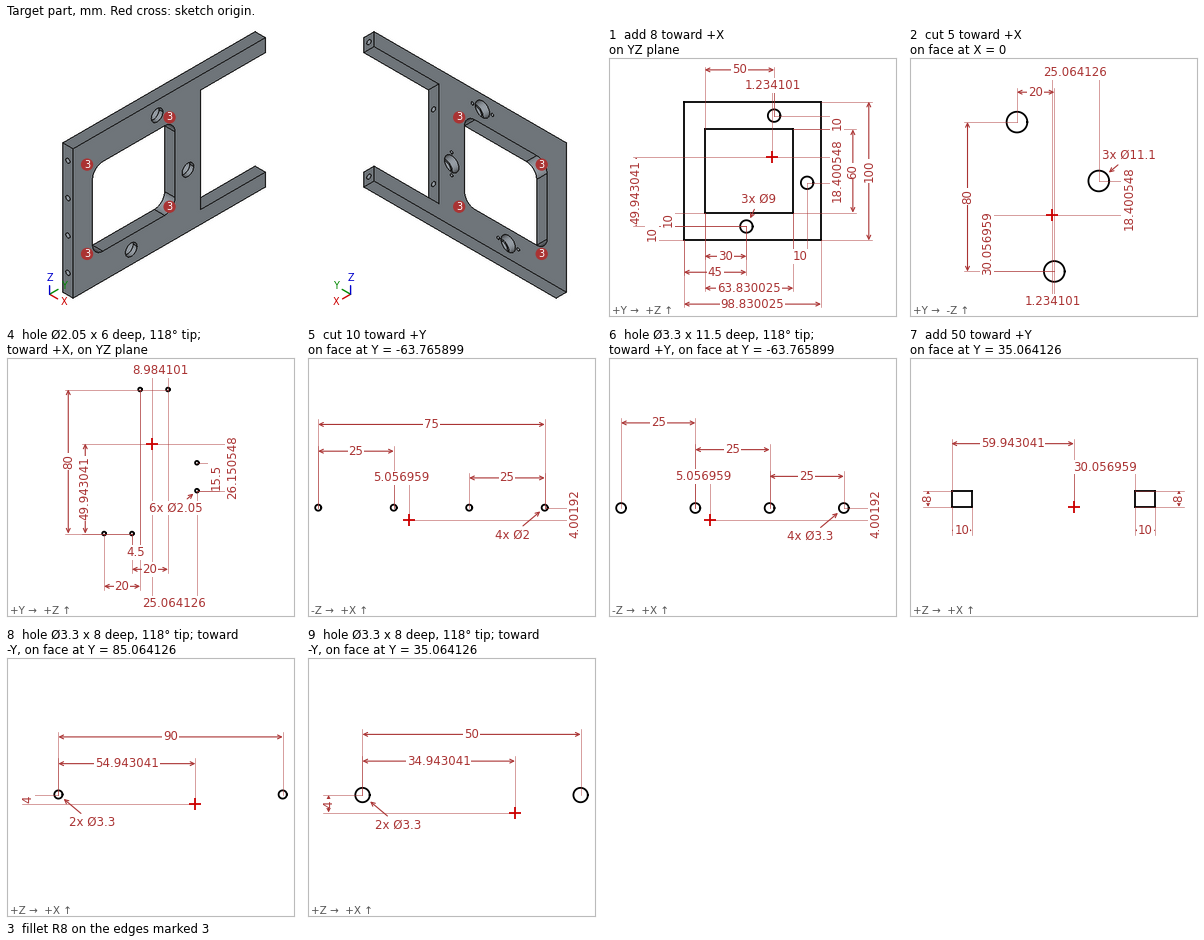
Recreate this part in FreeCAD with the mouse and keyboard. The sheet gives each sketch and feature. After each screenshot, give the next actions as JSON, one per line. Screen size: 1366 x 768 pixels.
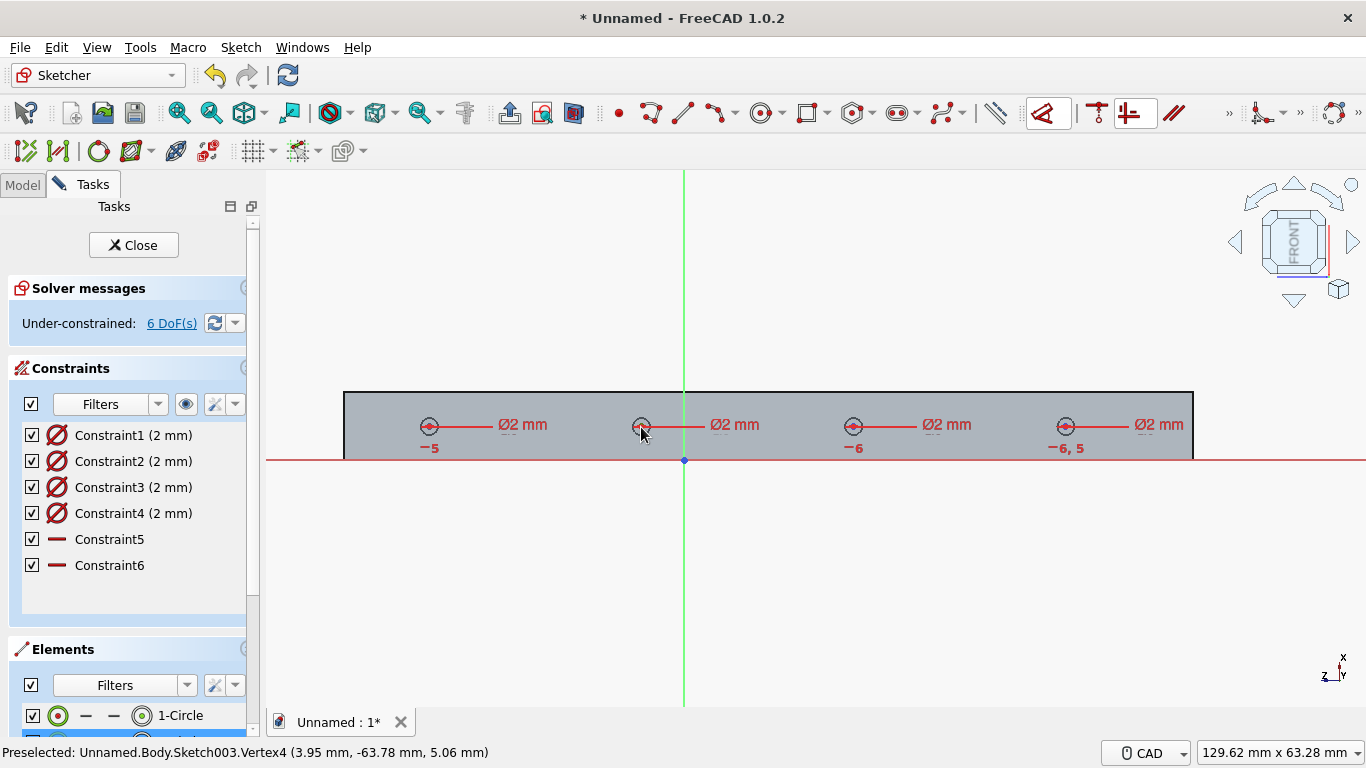
{"action": "left_click", "coordinate": [1152, 114]}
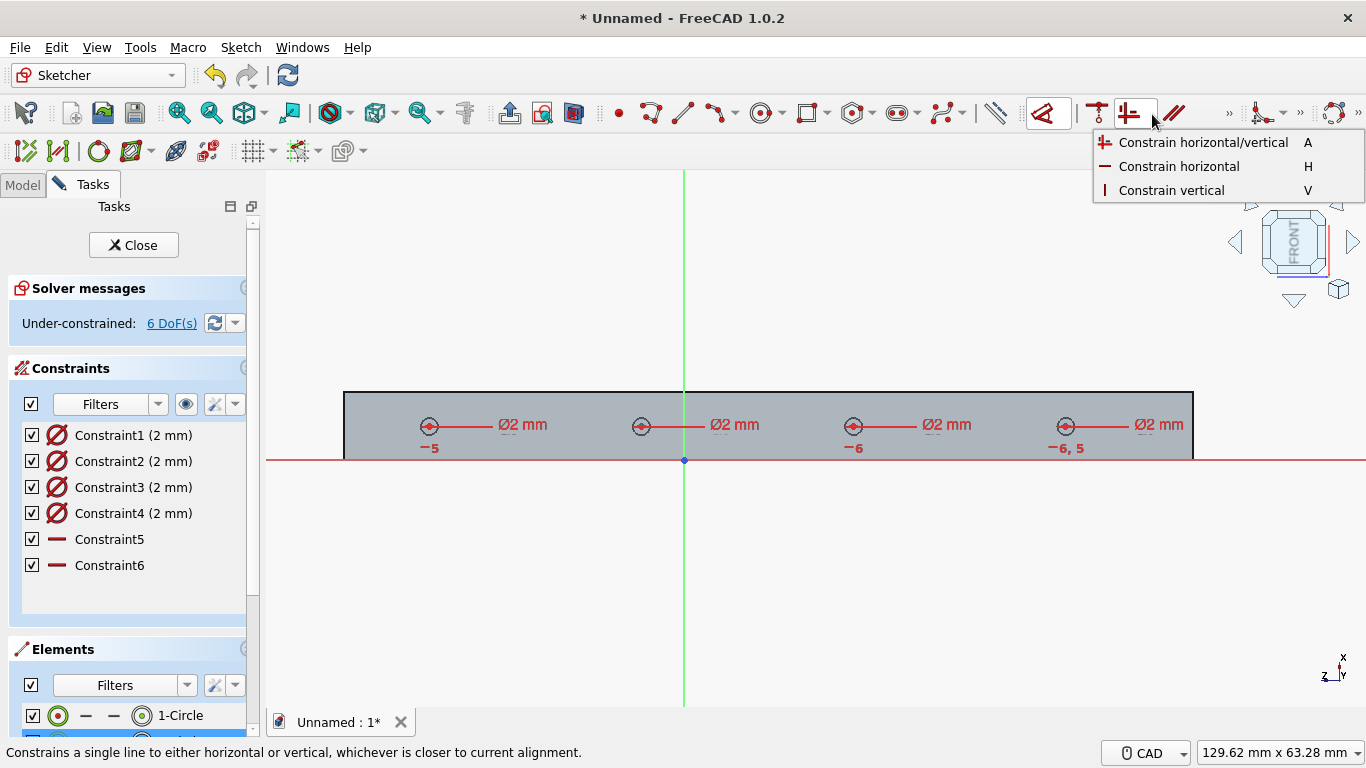
{"action": "left_click", "coordinate": [1229, 166]}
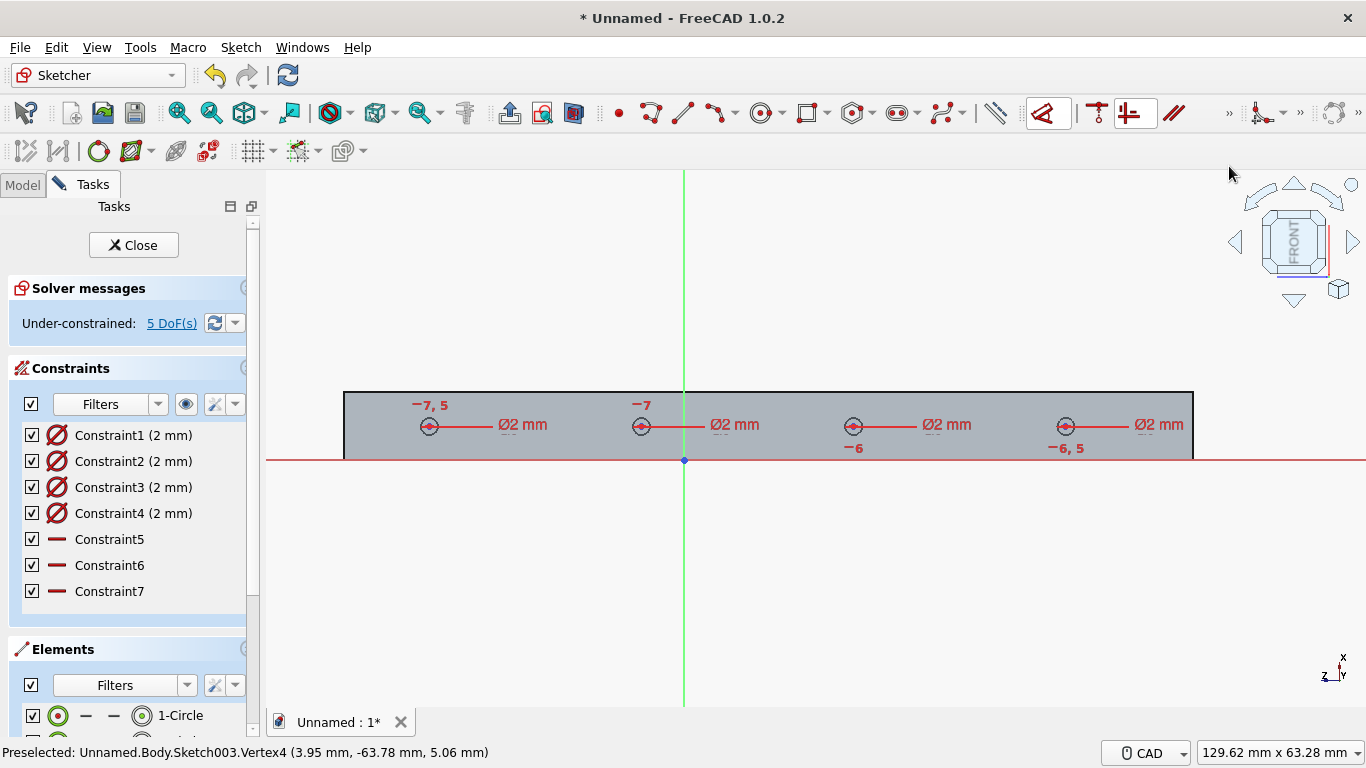
{"action": "left_click", "coordinate": [1066, 427]}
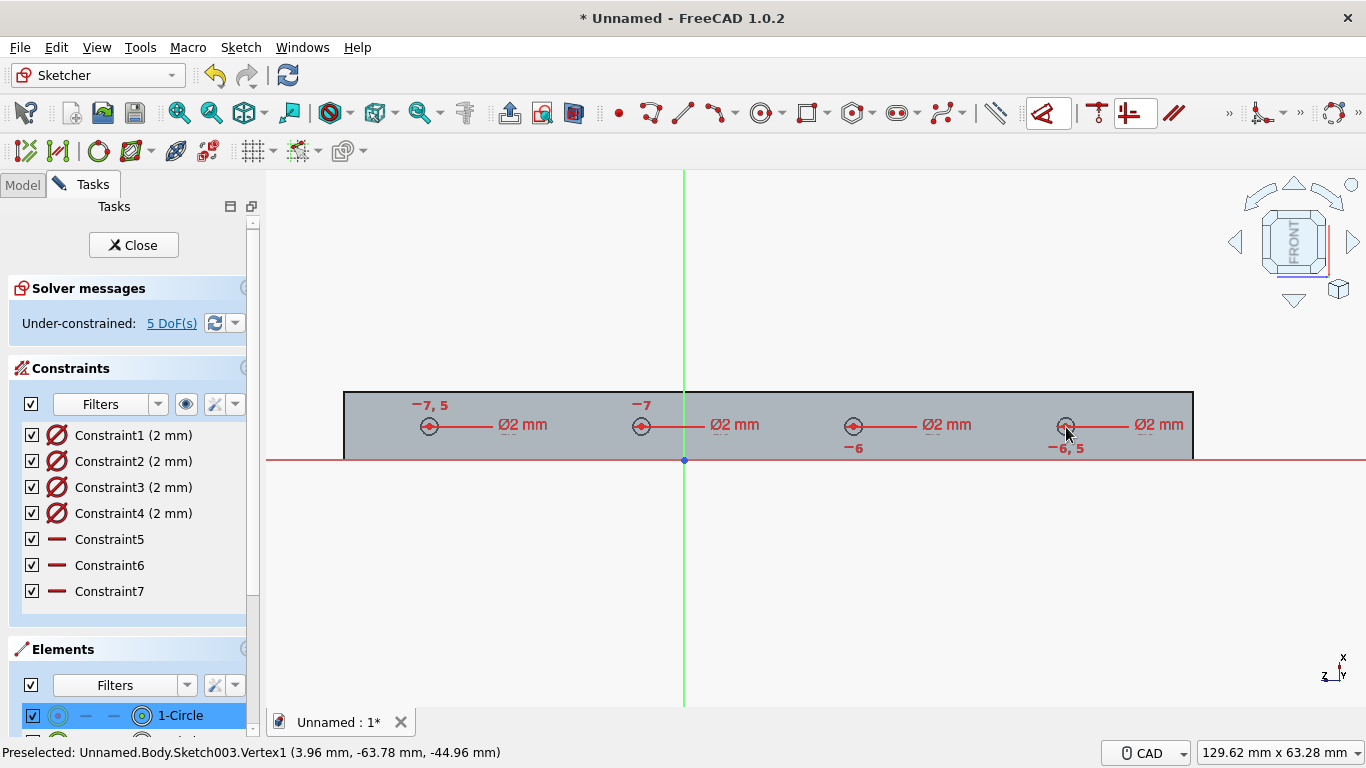
{"action": "left_click", "coordinate": [429, 427]}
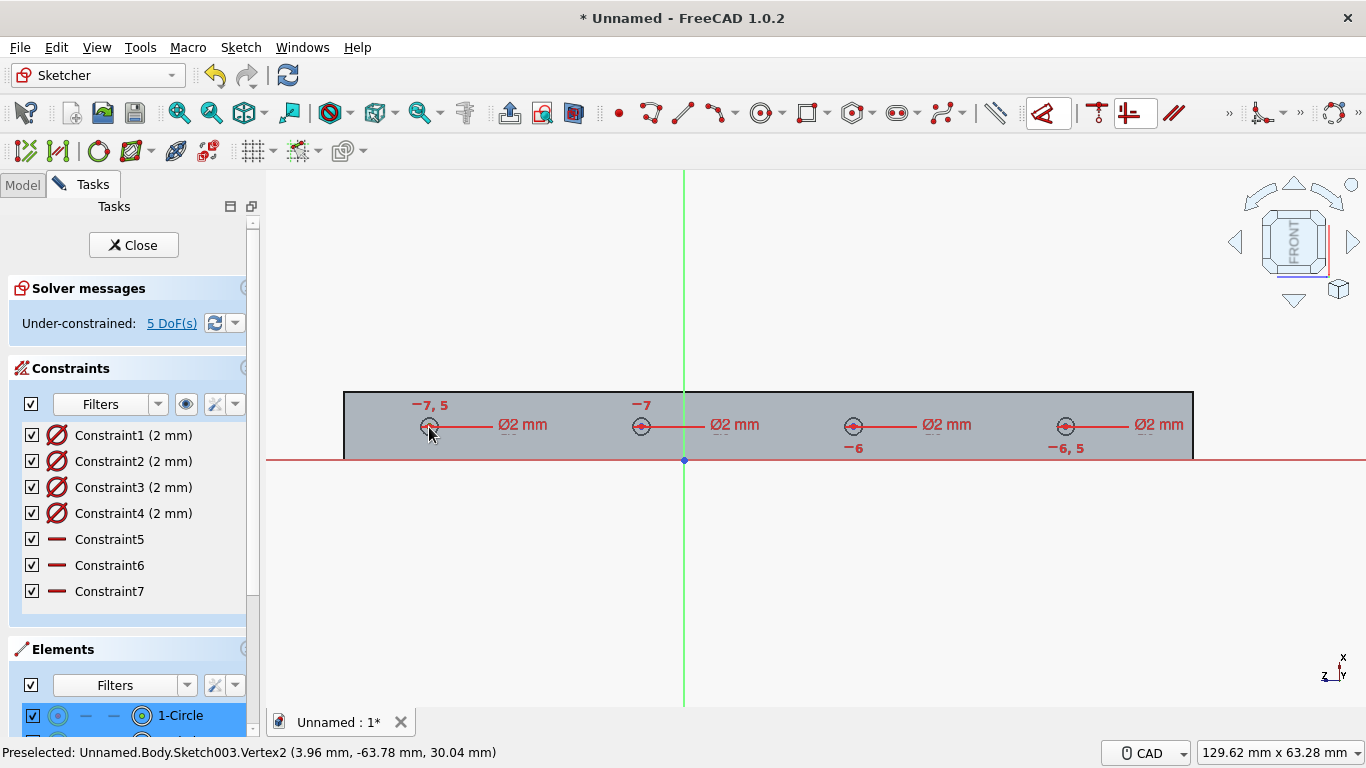
{"action": "key", "text": "l"}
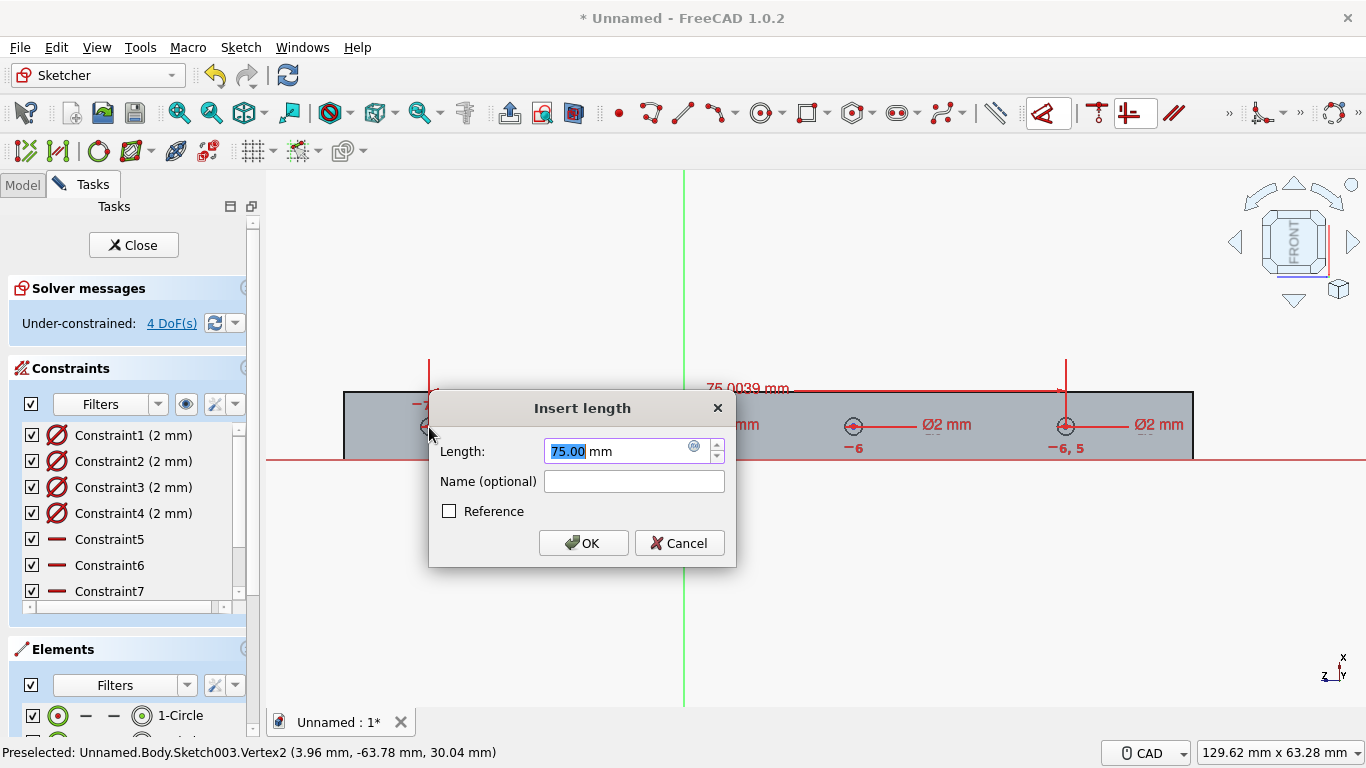
{"action": "type", "text": "75"}
{"action": "key", "text": "Return"}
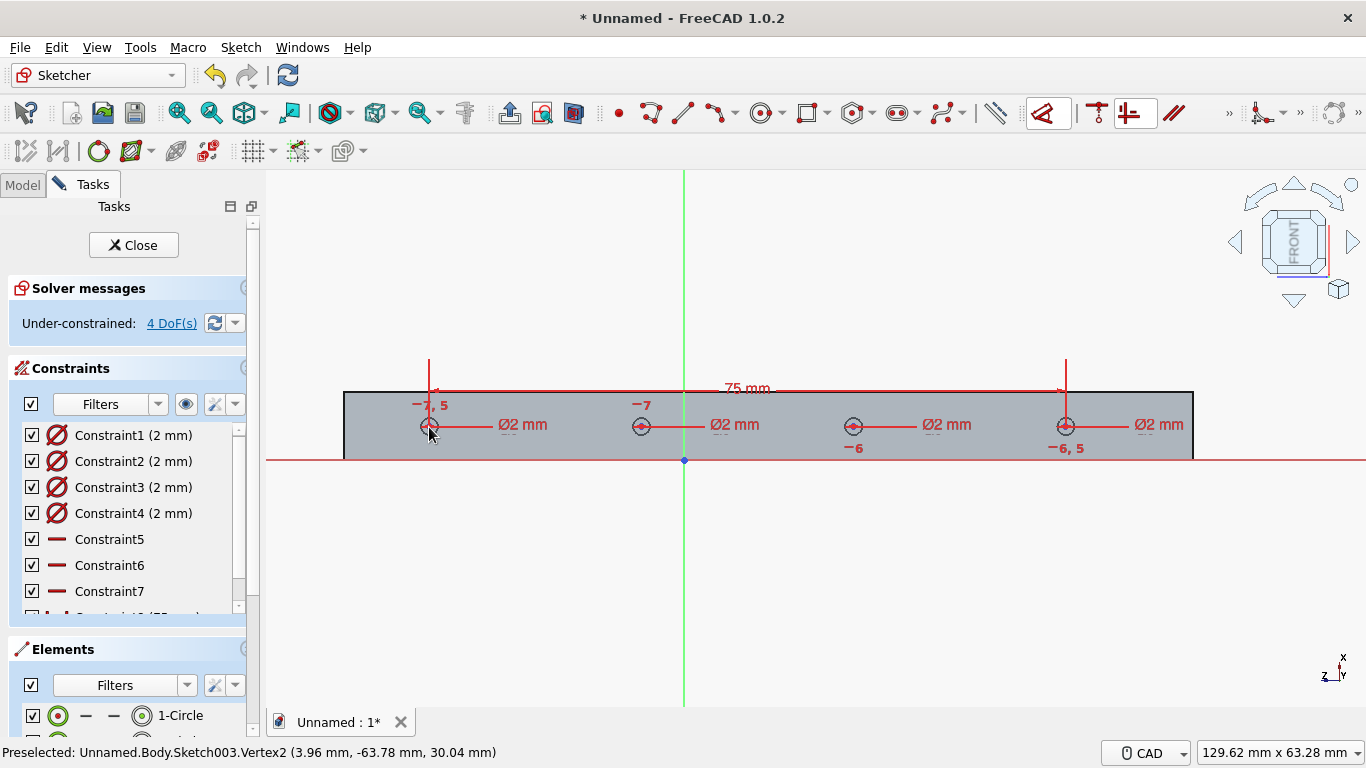
{"action": "left_click", "coordinate": [1066, 427]}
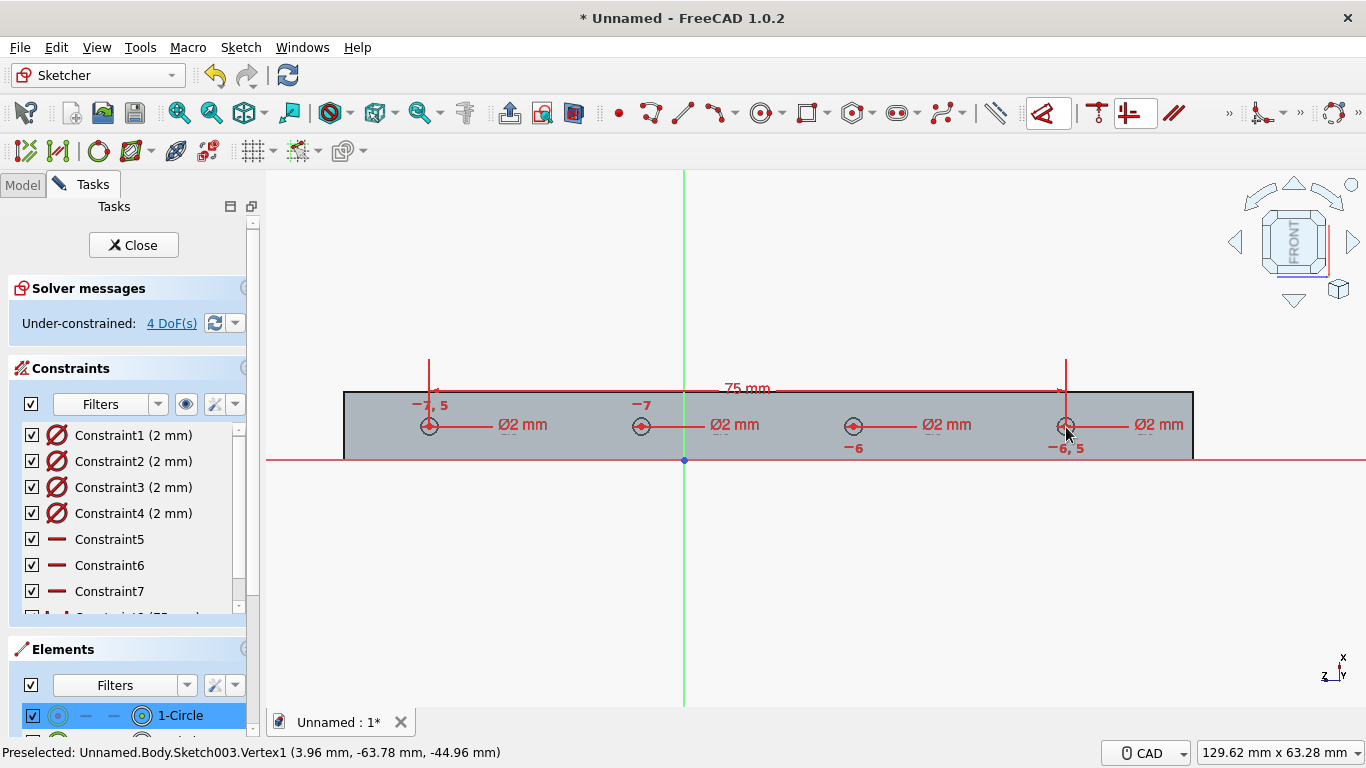
{"action": "left_click", "coordinate": [854, 427]}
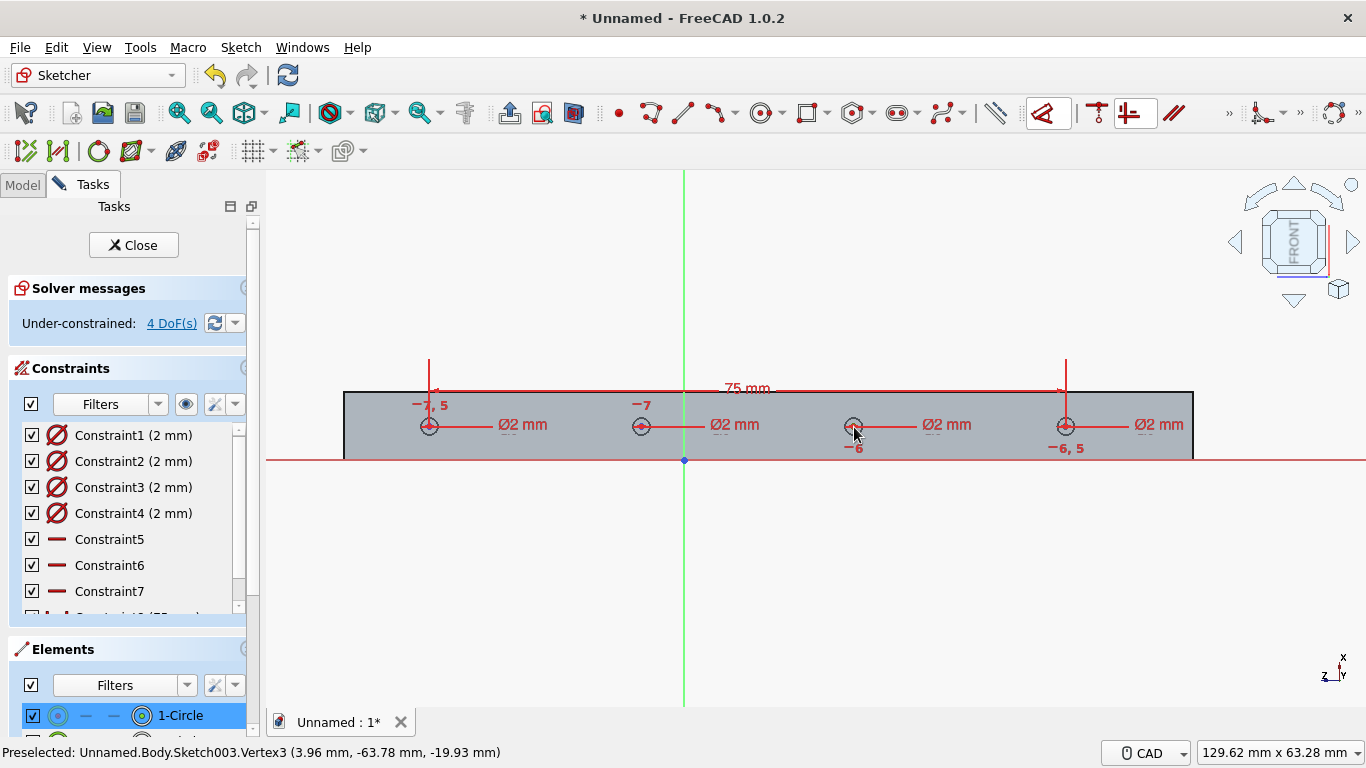
{"action": "key", "text": "l"}